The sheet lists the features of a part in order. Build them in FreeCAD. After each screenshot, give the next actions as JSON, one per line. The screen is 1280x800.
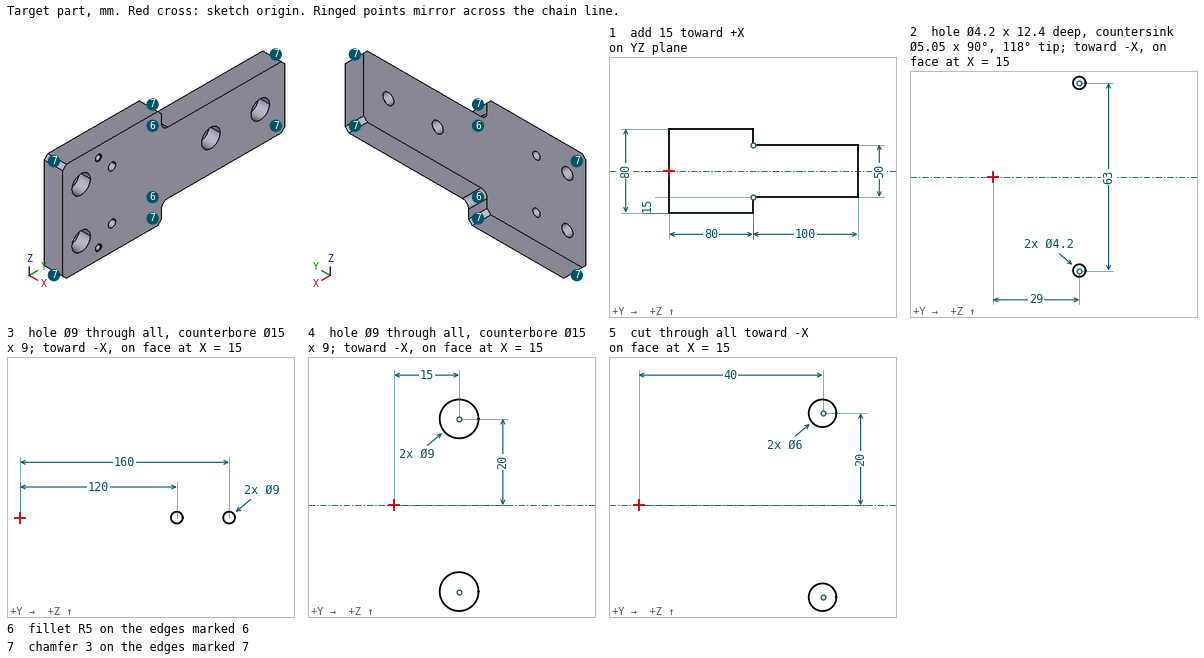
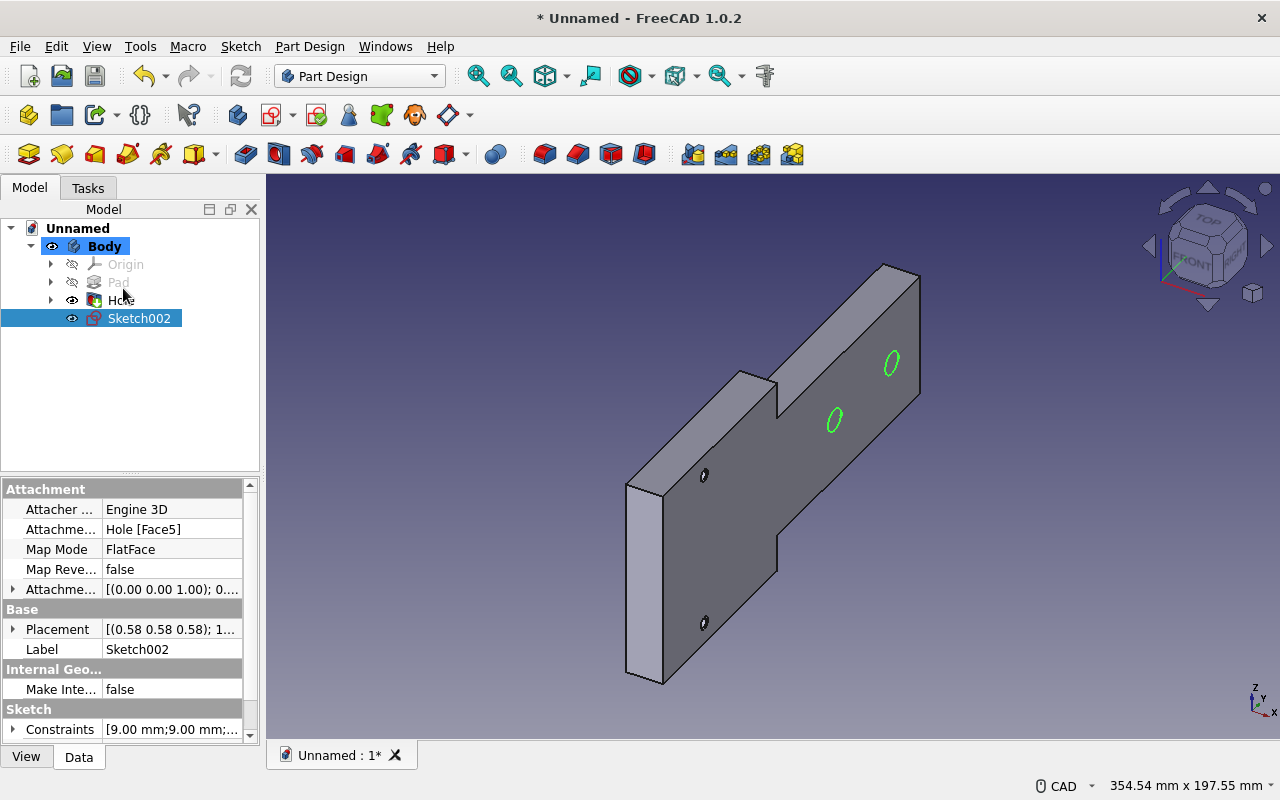
{"action": "left_click", "coordinate": [279, 154]}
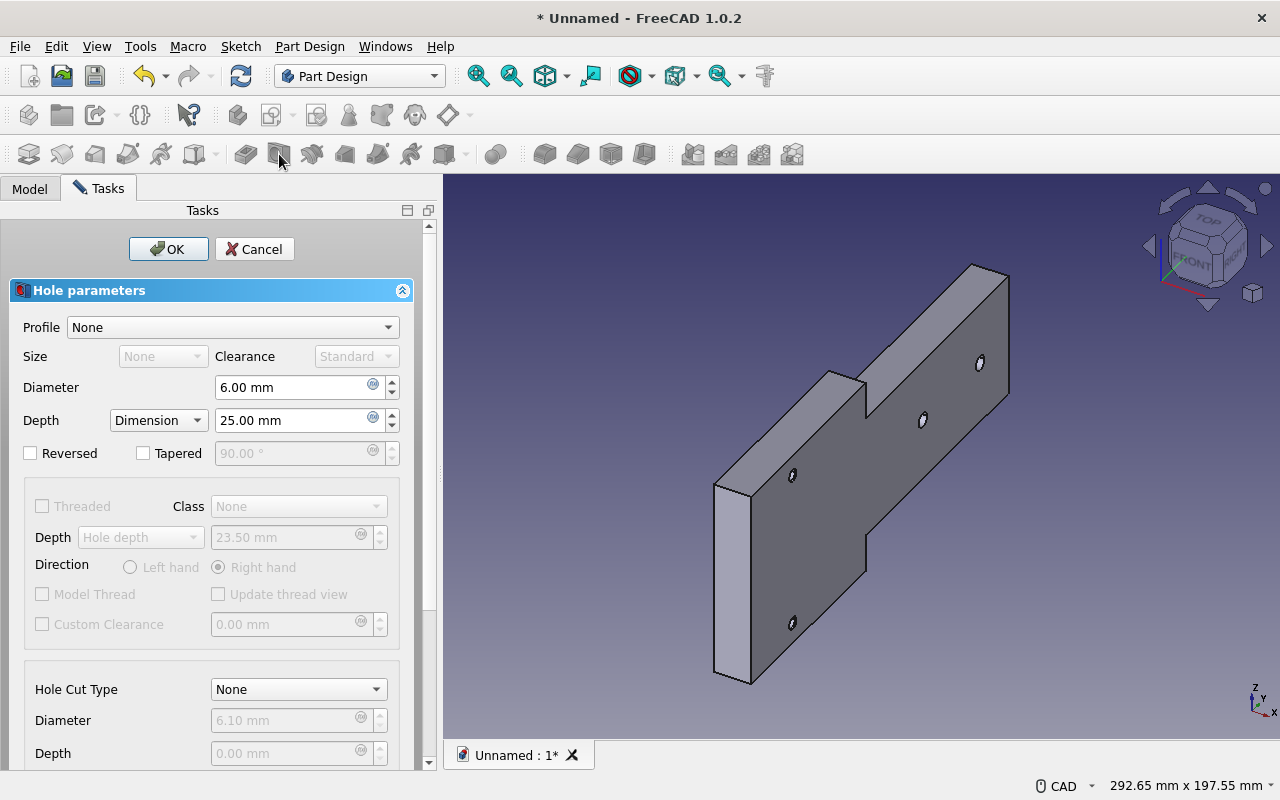
{"action": "triple_click", "coordinate": [300, 388]}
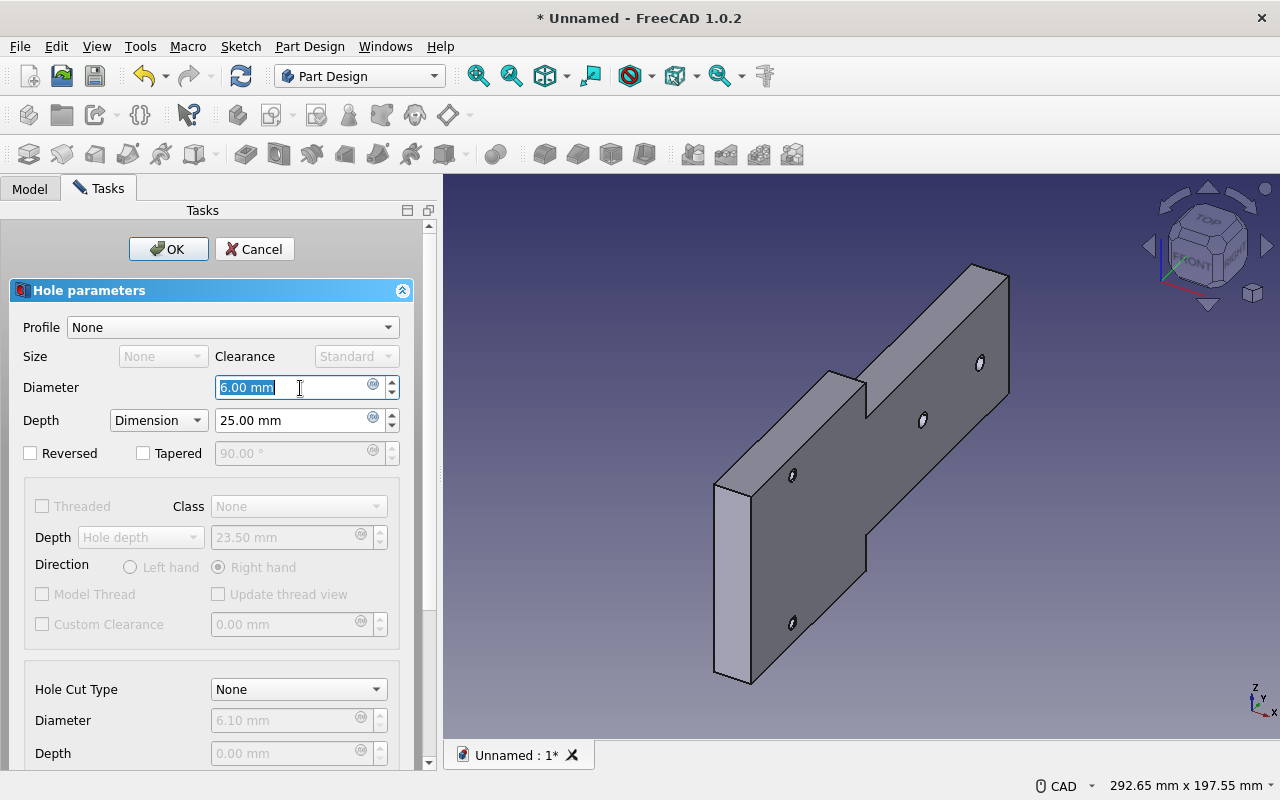
{"action": "type", "text": "9"}
{"action": "key", "text": "Tab"}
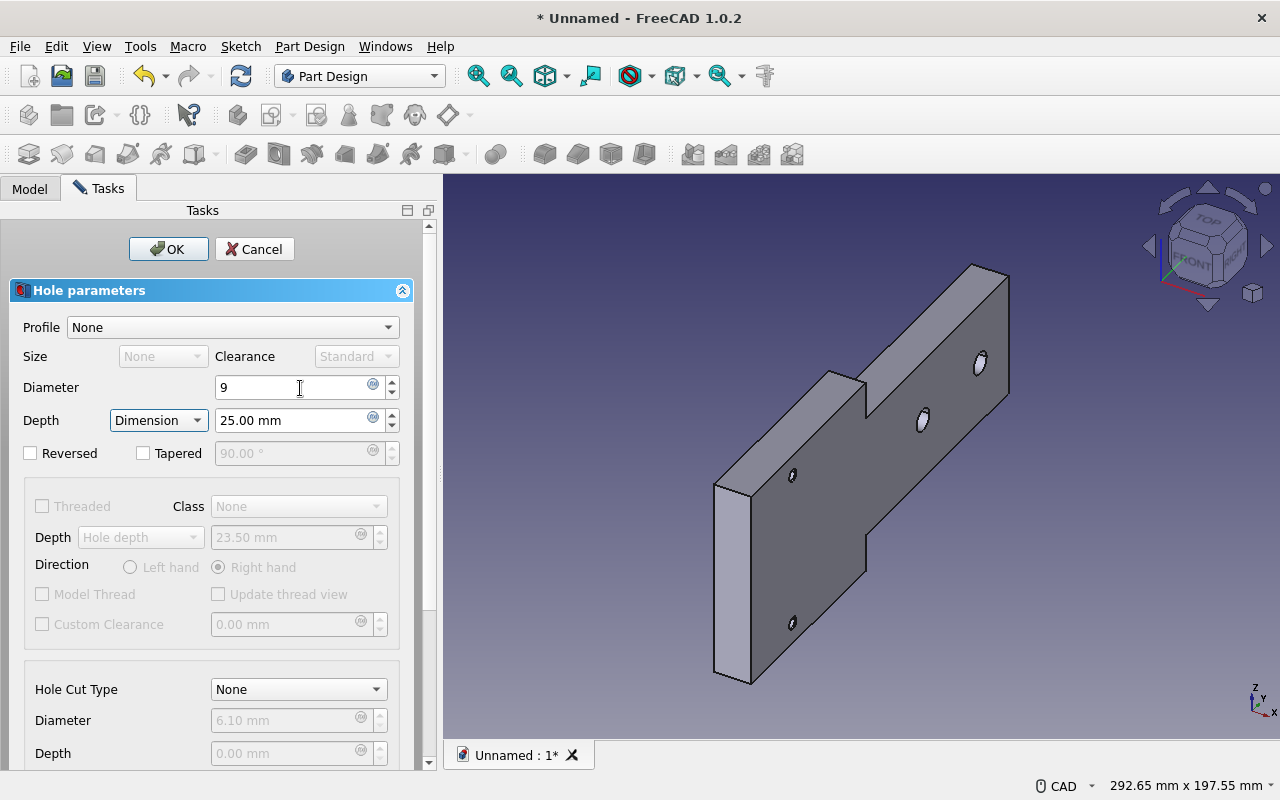
{"action": "left_click", "coordinate": [160, 420]}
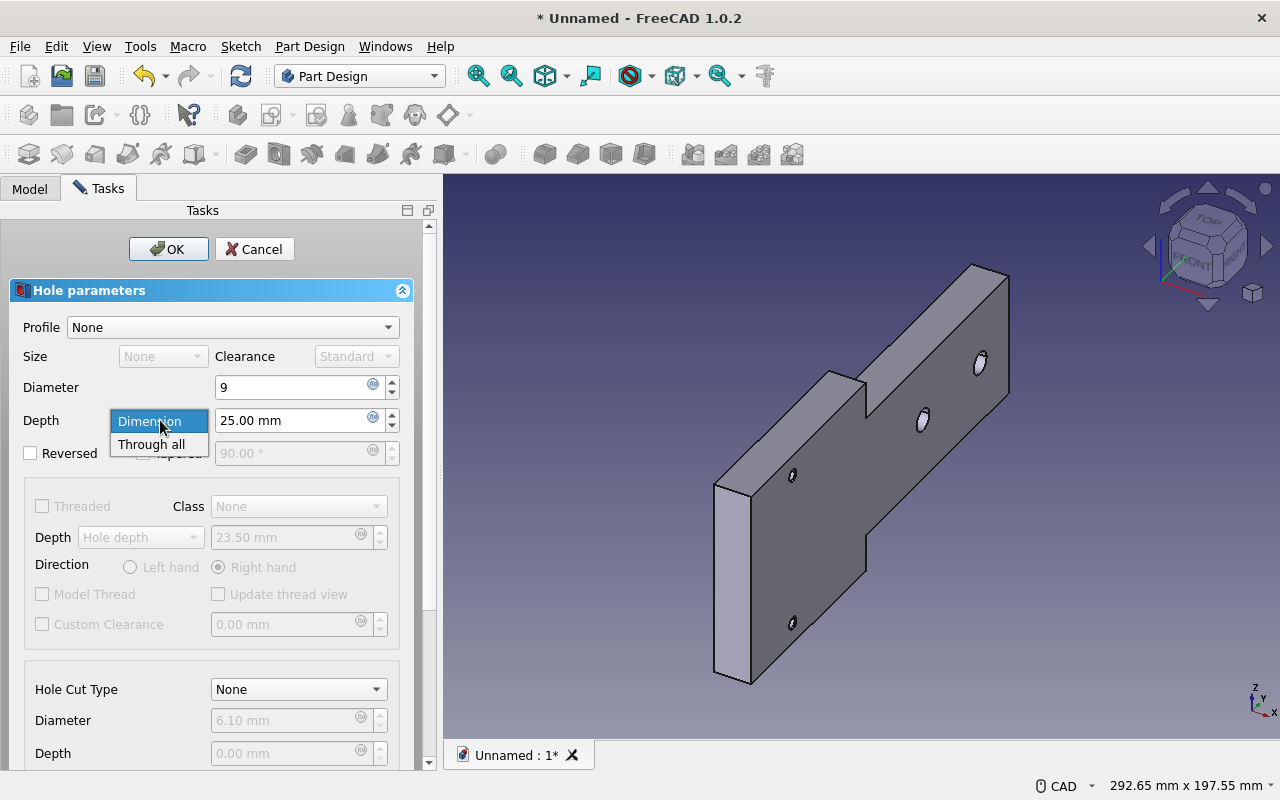
{"action": "left_click", "coordinate": [158, 444]}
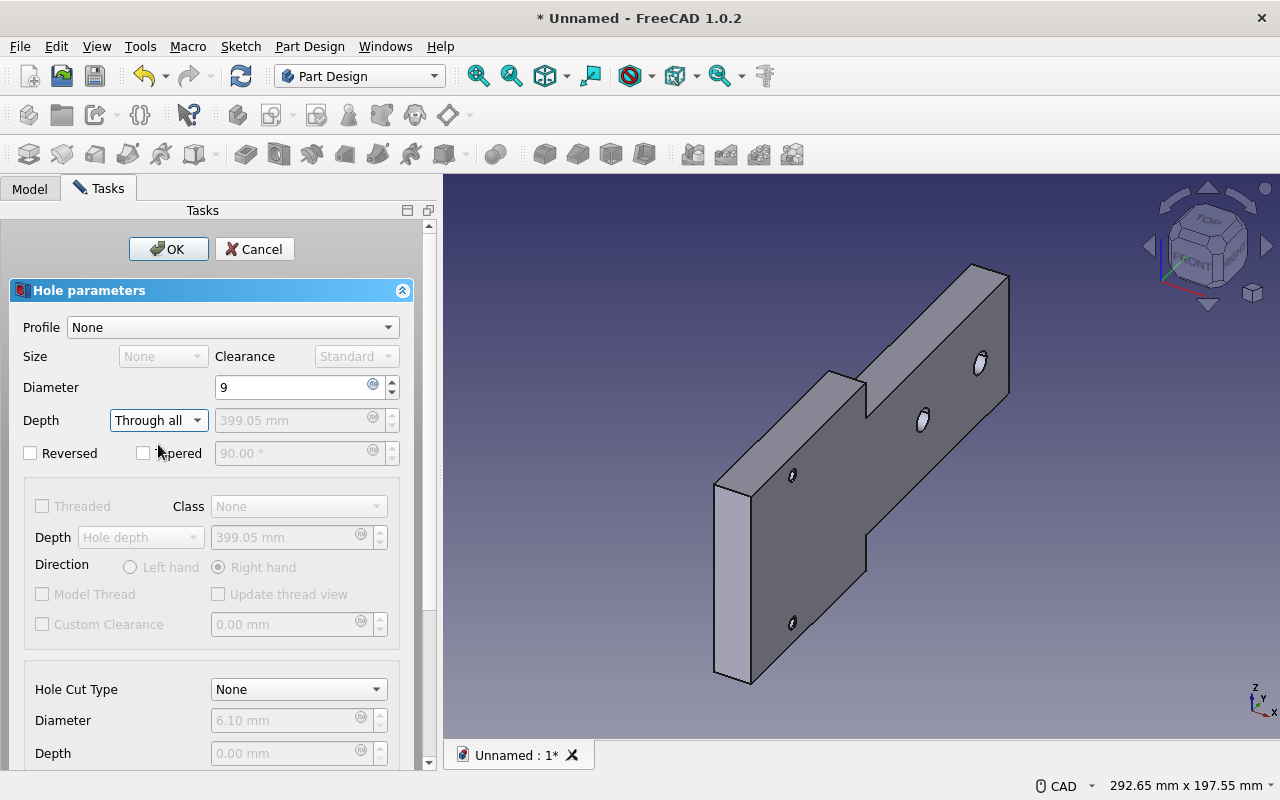
{"action": "left_click", "coordinate": [300, 690]}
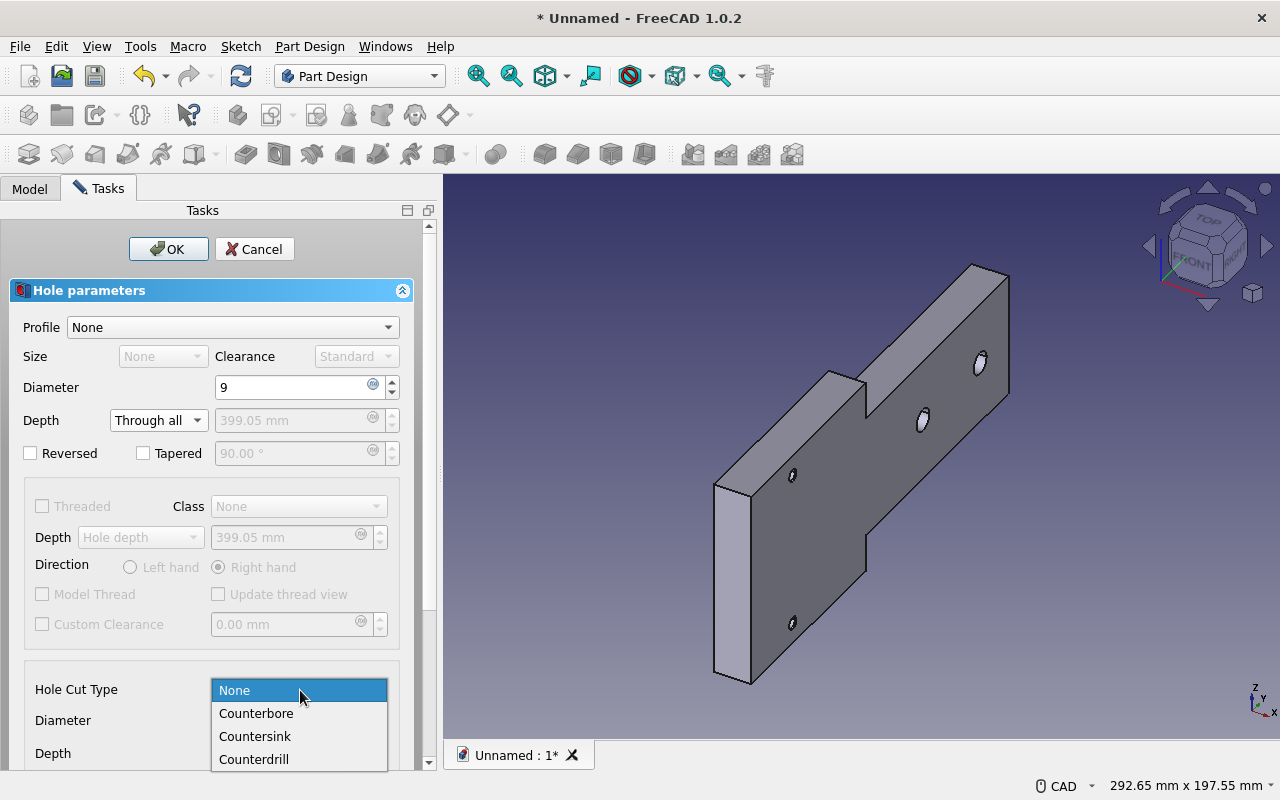
{"action": "left_click", "coordinate": [298, 714]}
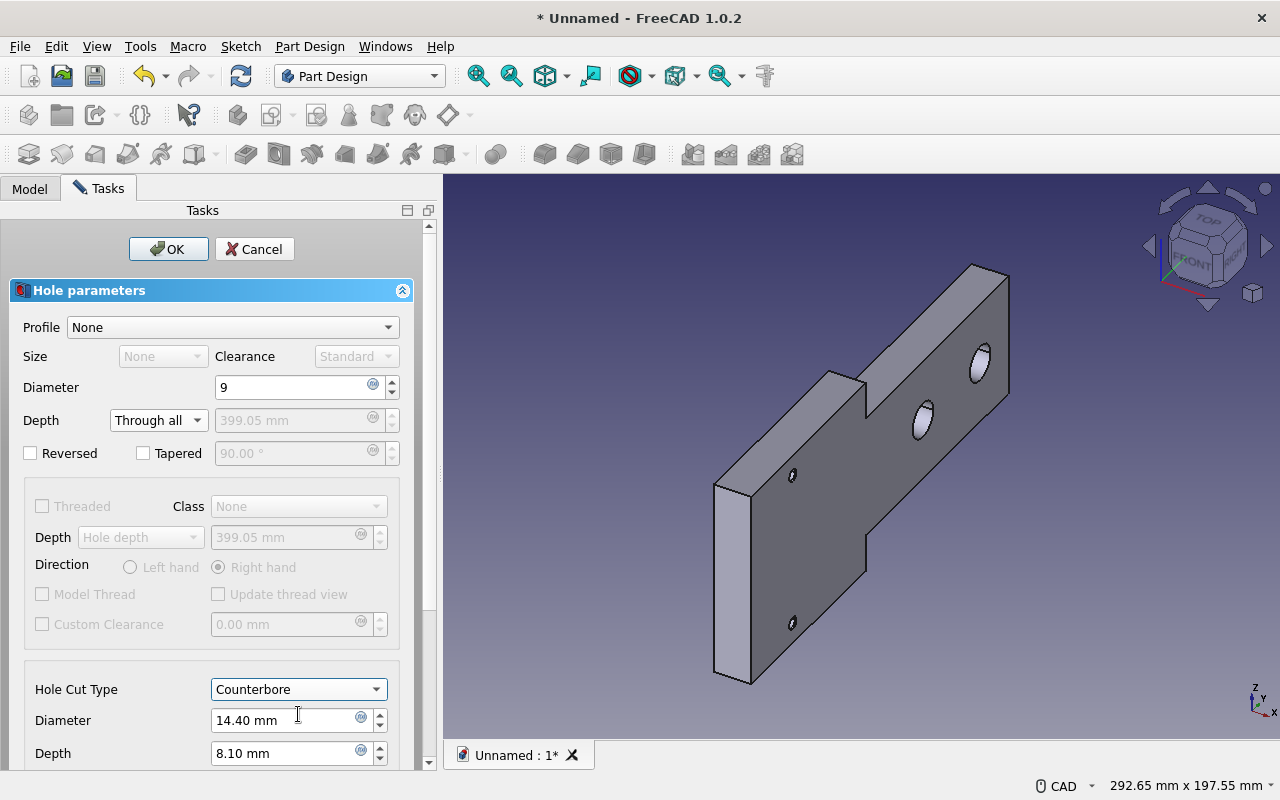
{"action": "triple_click", "coordinate": [292, 720]}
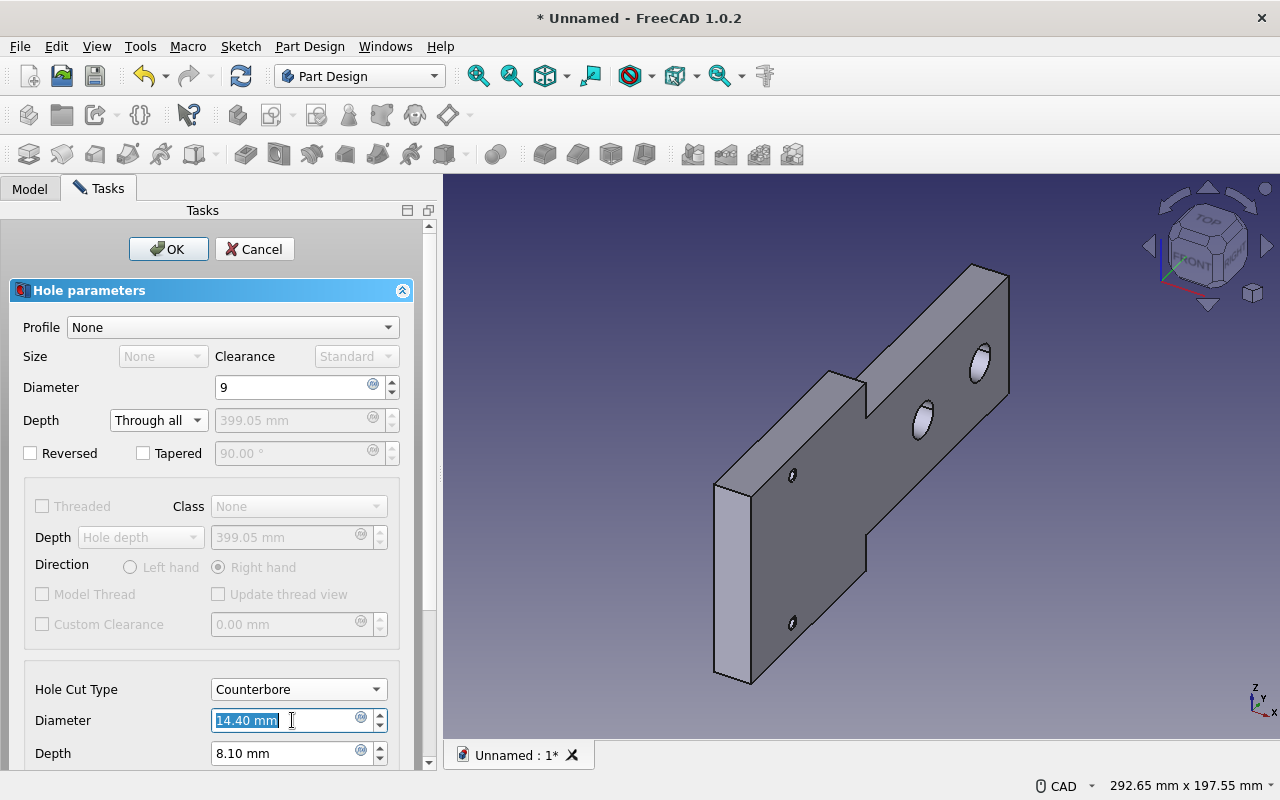
{"action": "type", "text": "15"}
{"action": "key", "text": "Tab"}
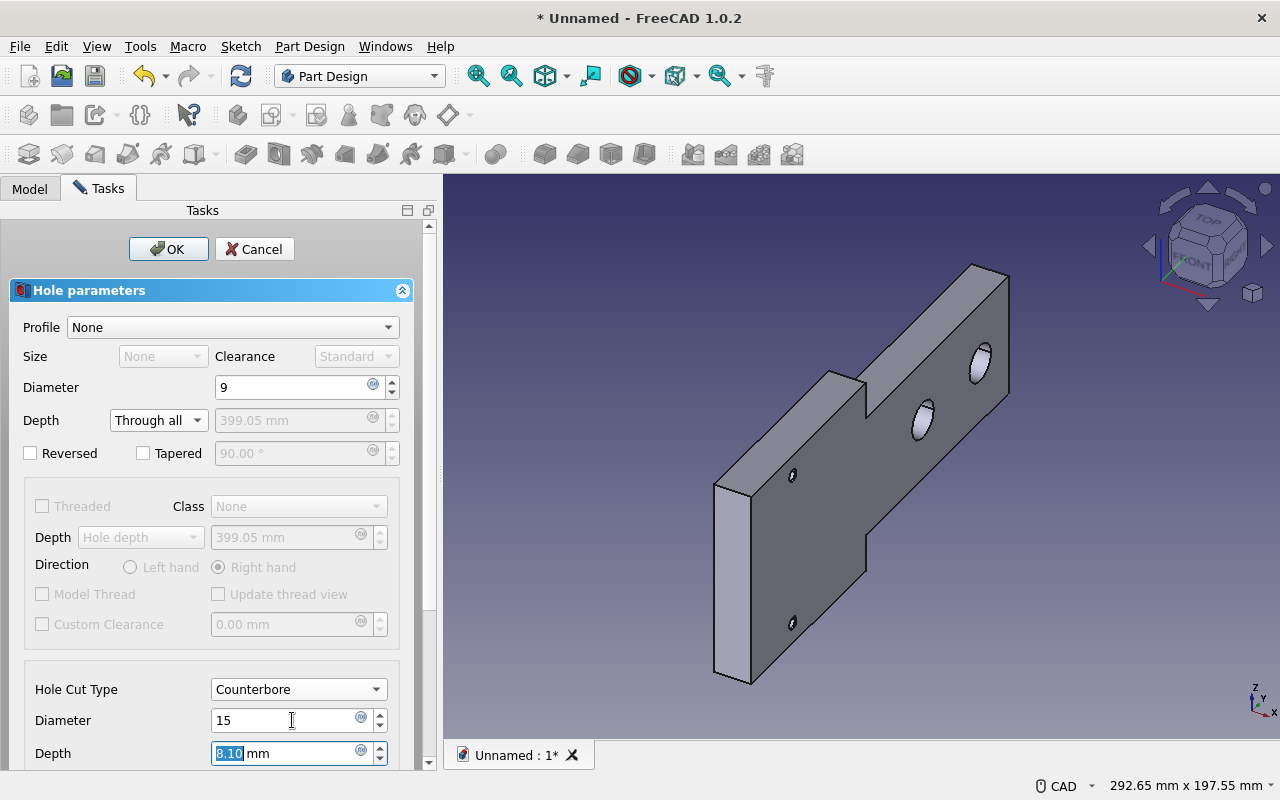
{"action": "type", "text": "9"}
{"action": "key", "text": "Tab"}